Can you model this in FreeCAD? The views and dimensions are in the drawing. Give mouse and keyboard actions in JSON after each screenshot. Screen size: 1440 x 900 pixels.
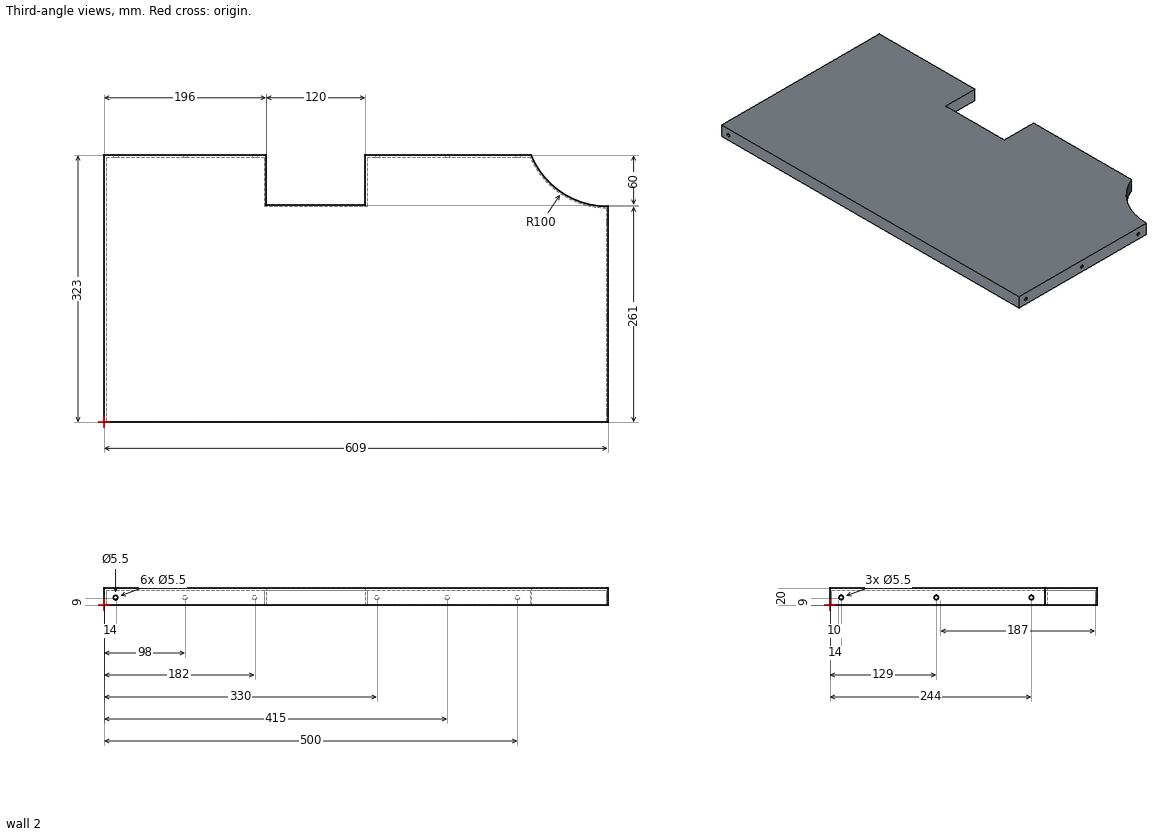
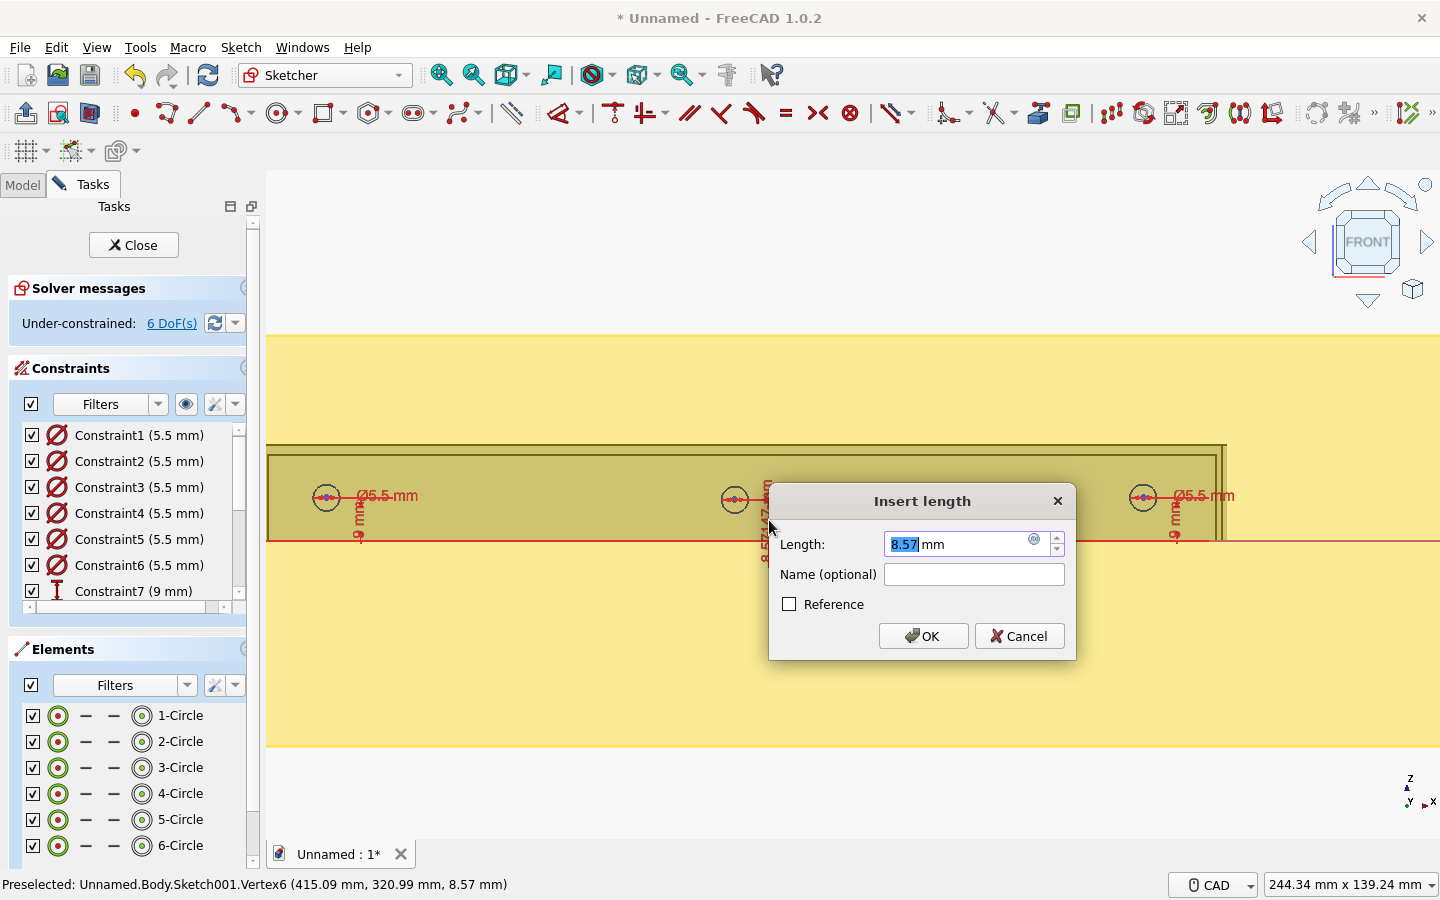
{"action": "type", "text": "9"}
{"action": "key", "text": "Return"}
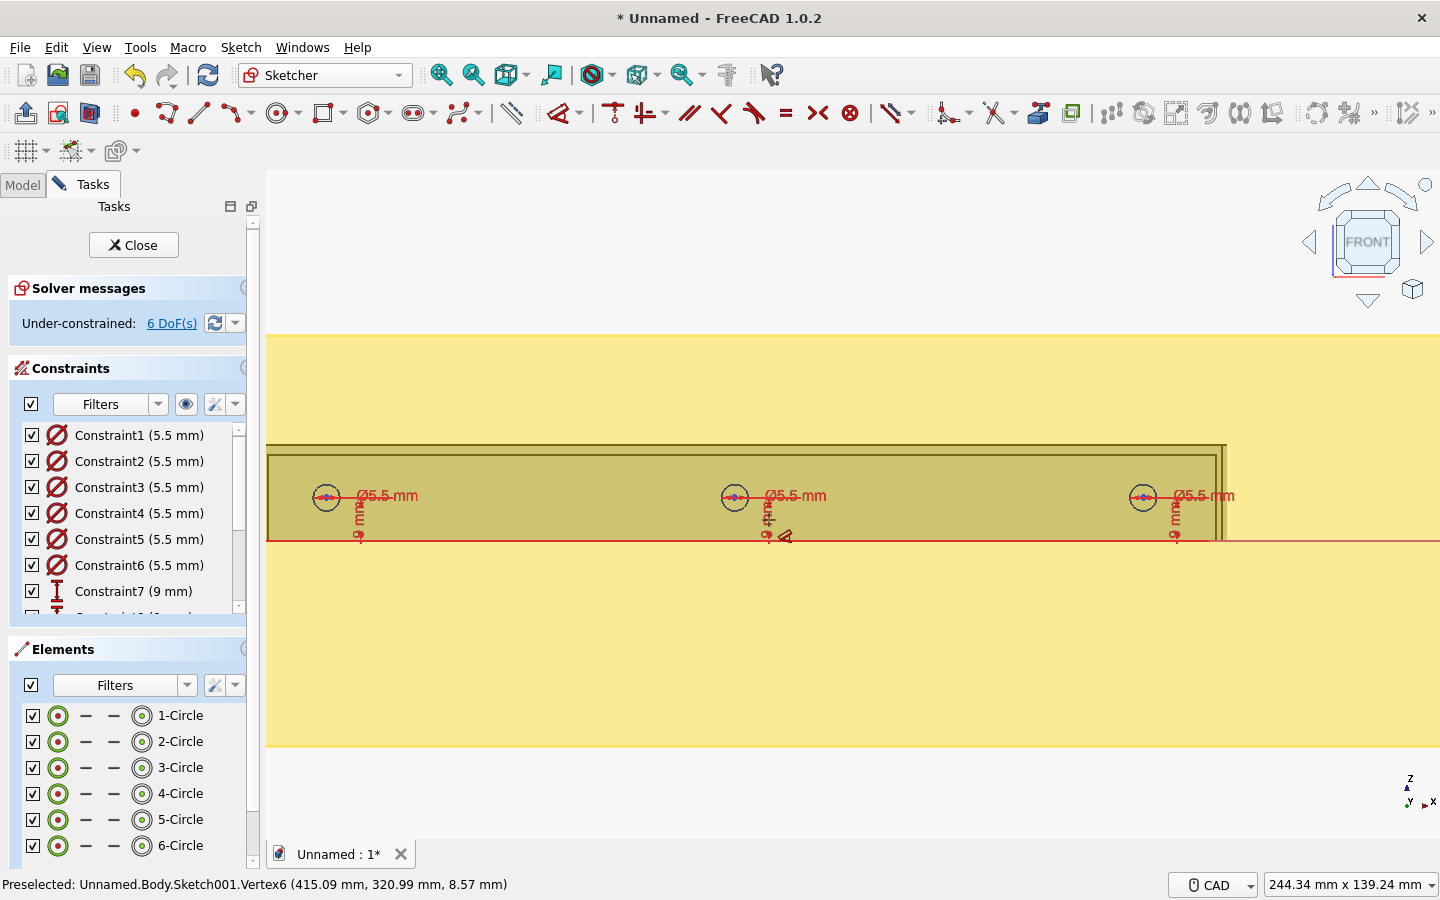
{"action": "scroll", "coordinate": [1145, 501], "scroll_direction": "down", "scroll_amount": 6}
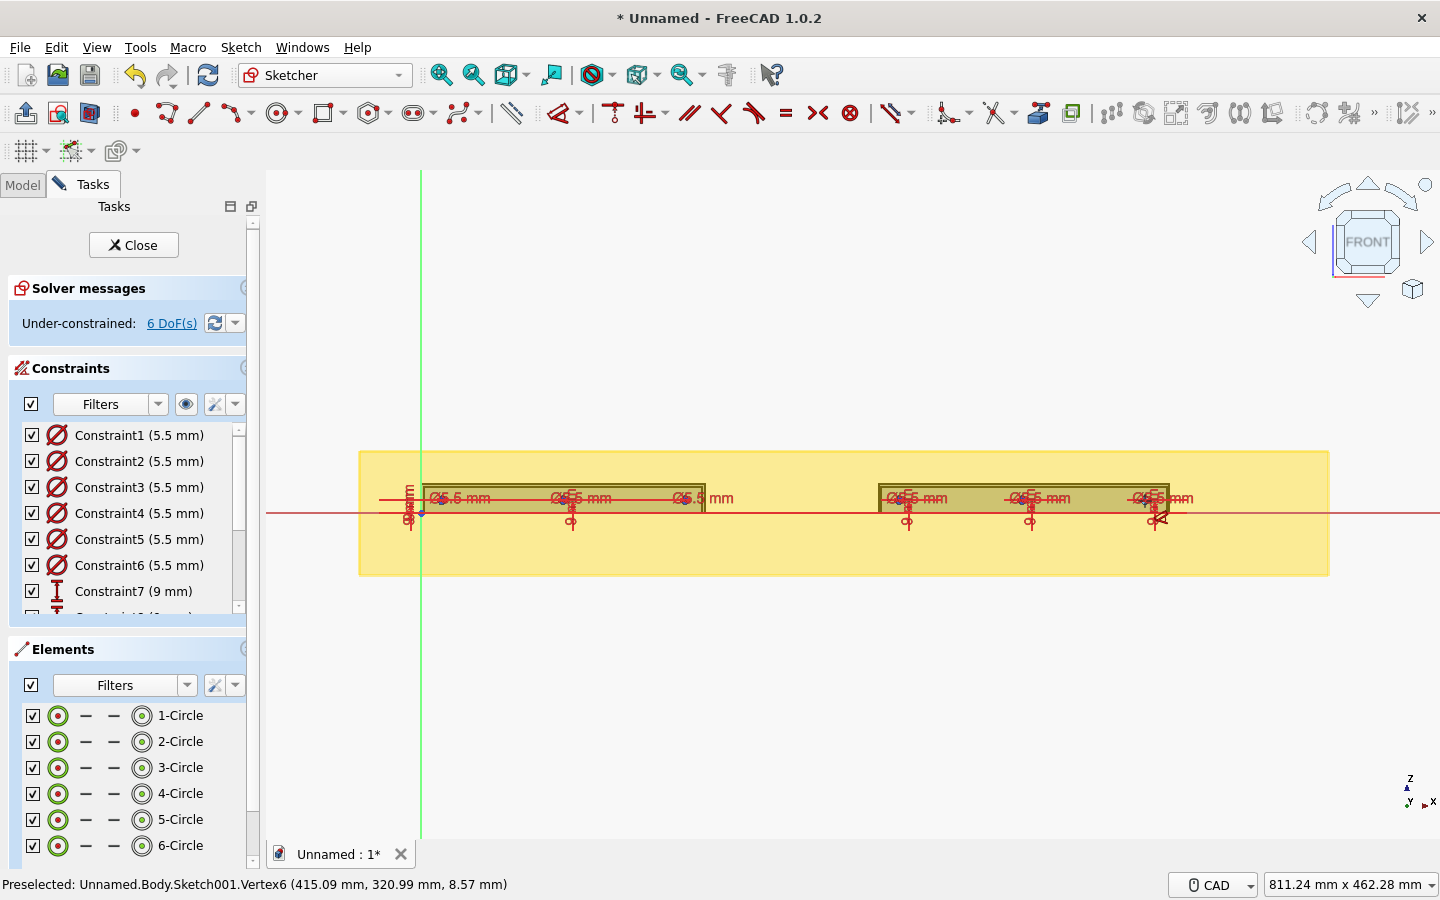
{"action": "scroll", "coordinate": [442, 500], "scroll_direction": "up", "scroll_amount": 4}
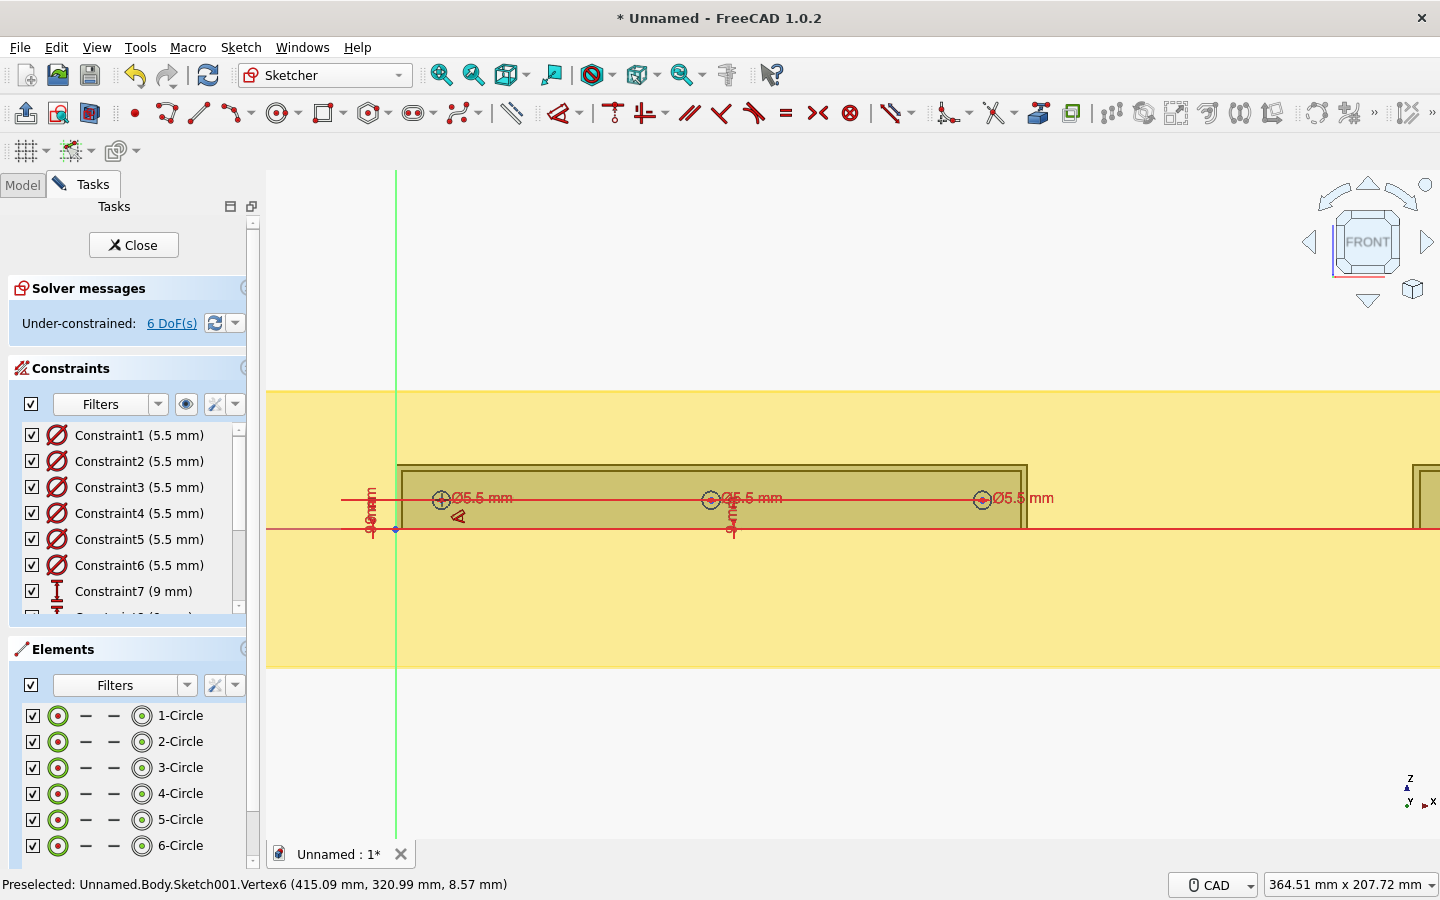
{"action": "left_click", "coordinate": [441, 500]}
{"action": "left_click", "coordinate": [419, 563]}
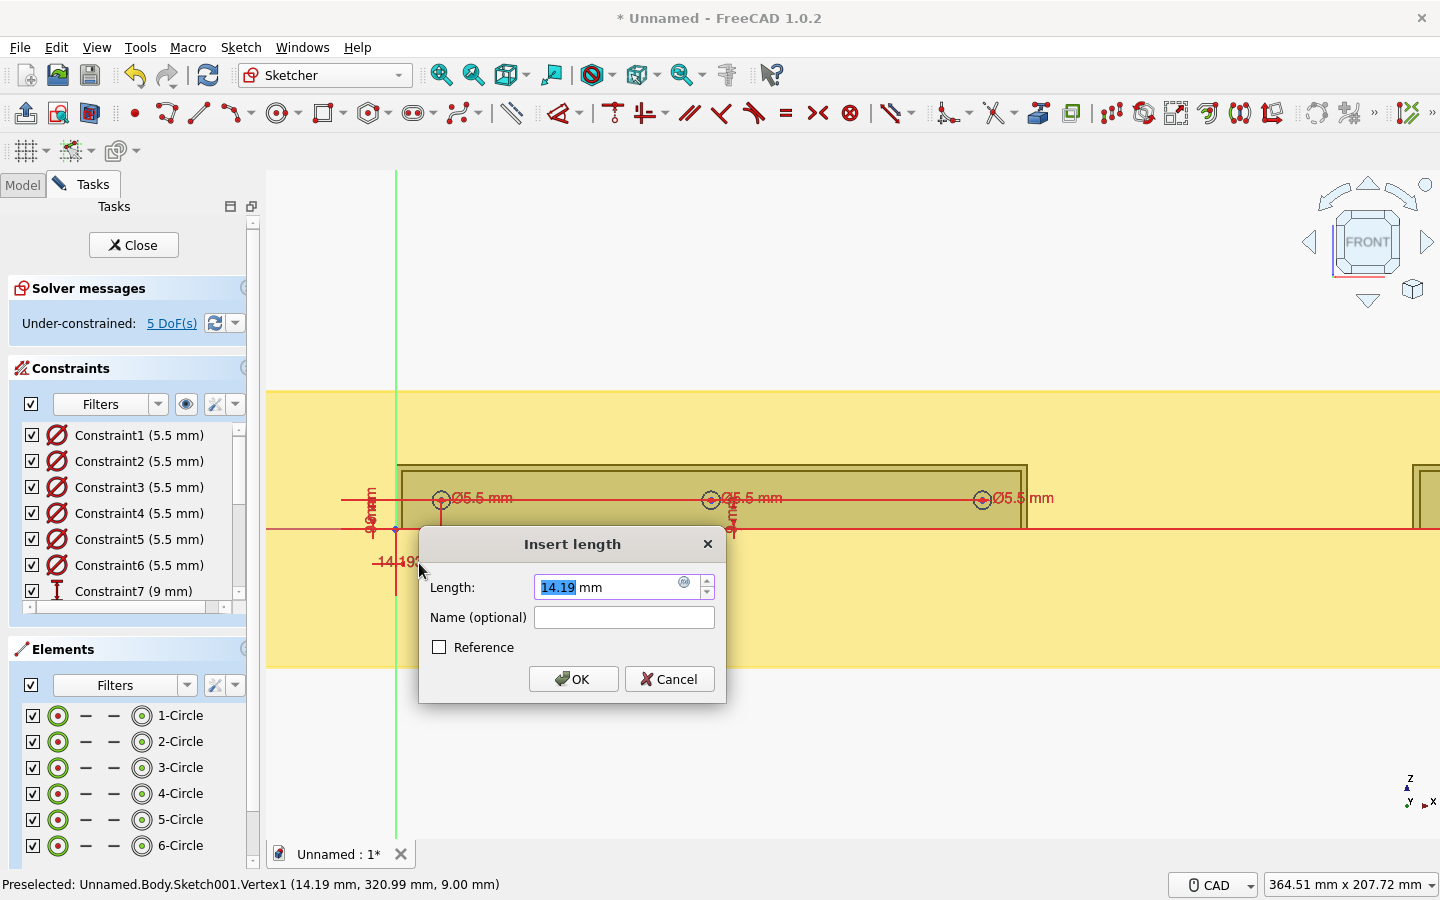
{"action": "type", "text": "14"}
{"action": "key", "text": "Return"}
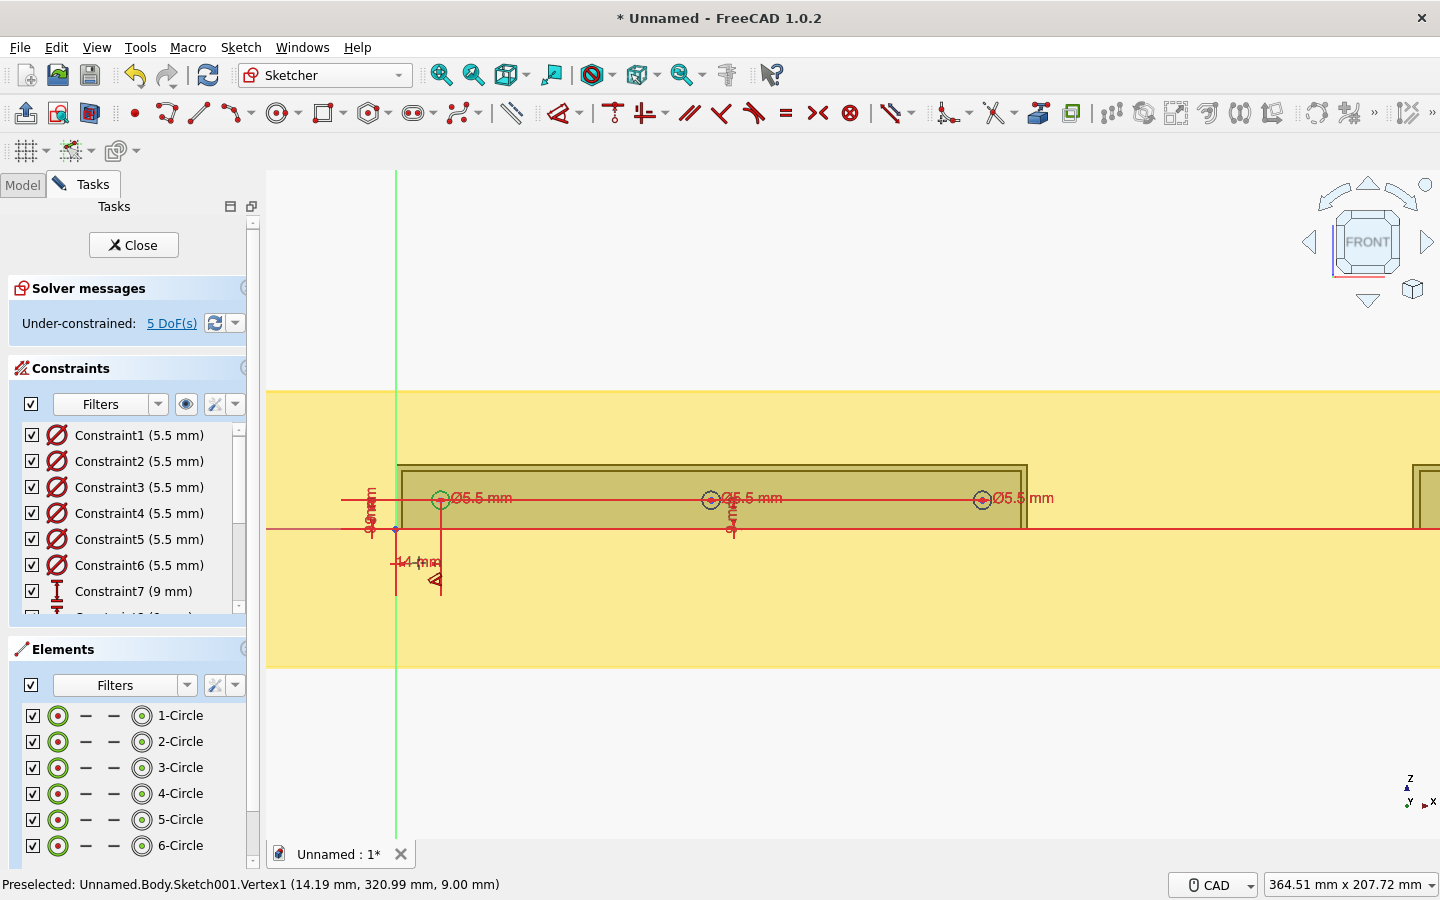
{"action": "left_click", "coordinate": [711, 500]}
{"action": "left_click", "coordinate": [553, 563]}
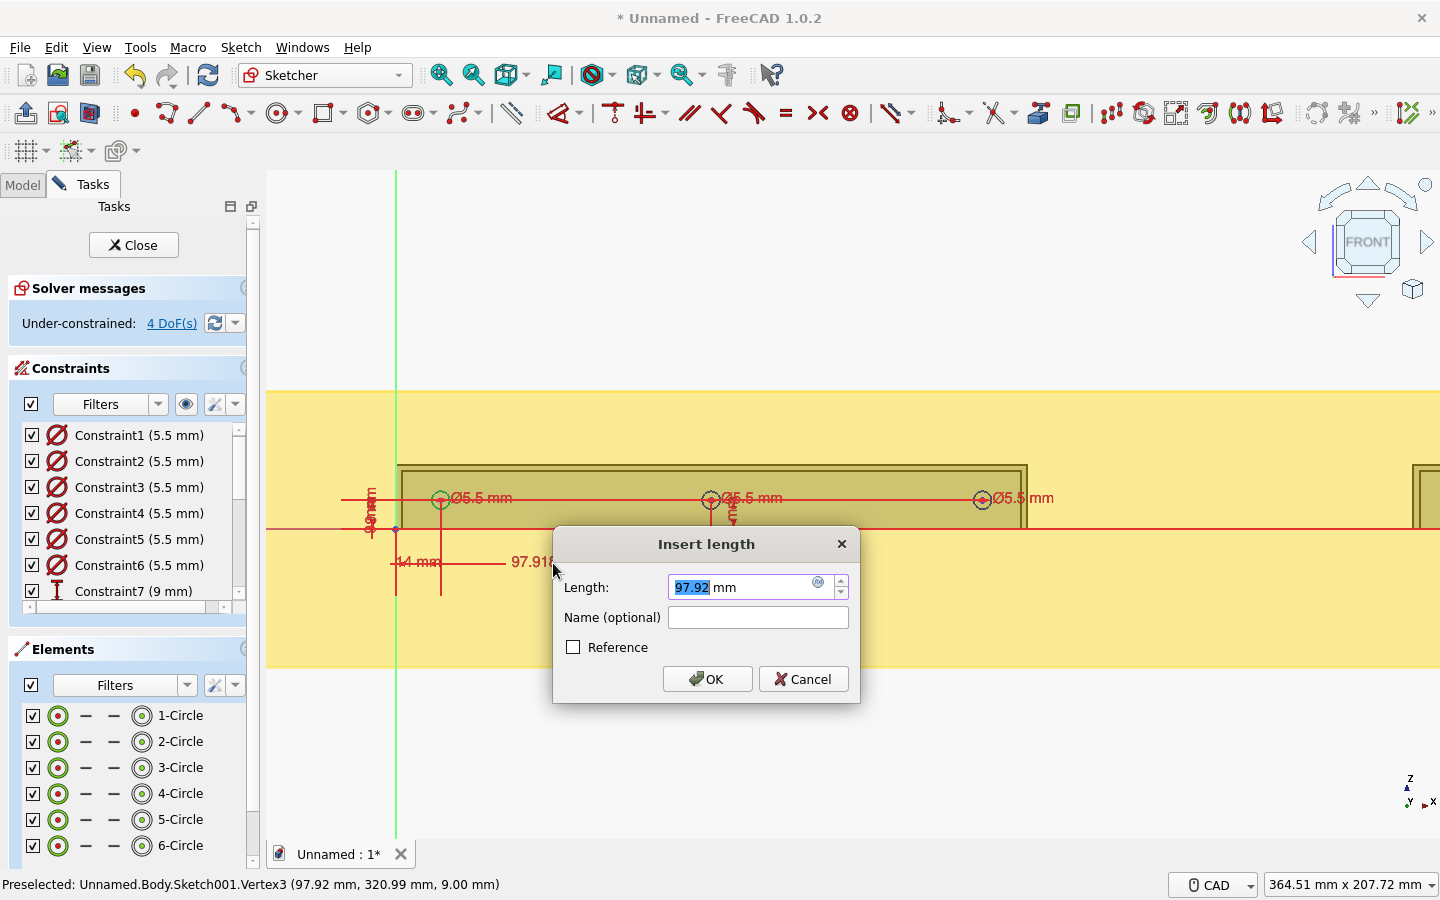
{"action": "type", "text": "98"}
{"action": "key", "text": "Return"}